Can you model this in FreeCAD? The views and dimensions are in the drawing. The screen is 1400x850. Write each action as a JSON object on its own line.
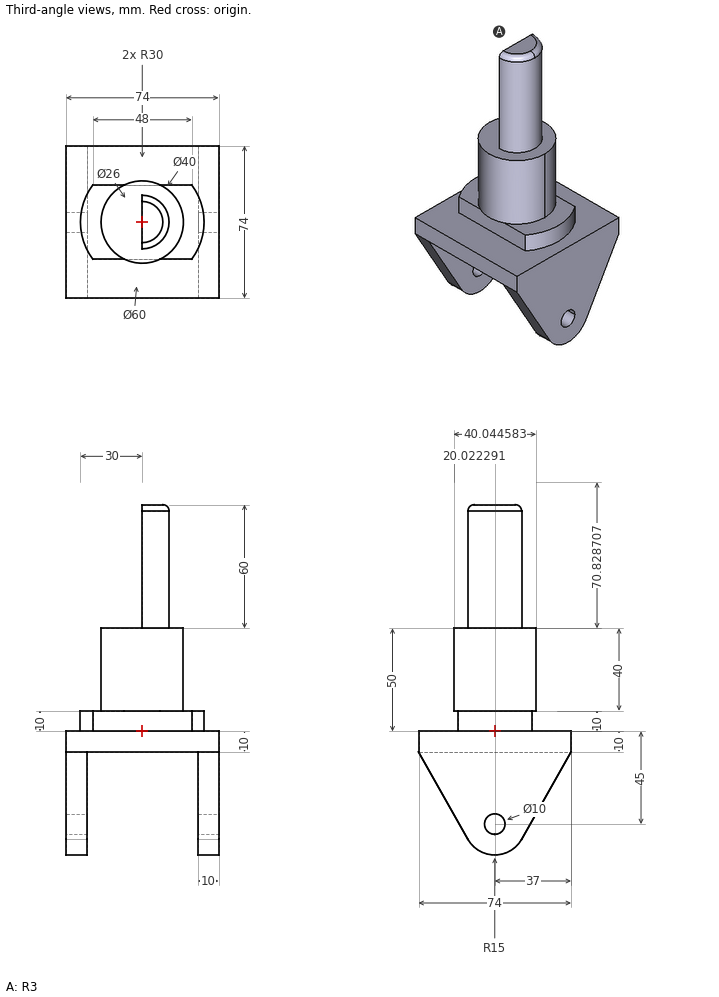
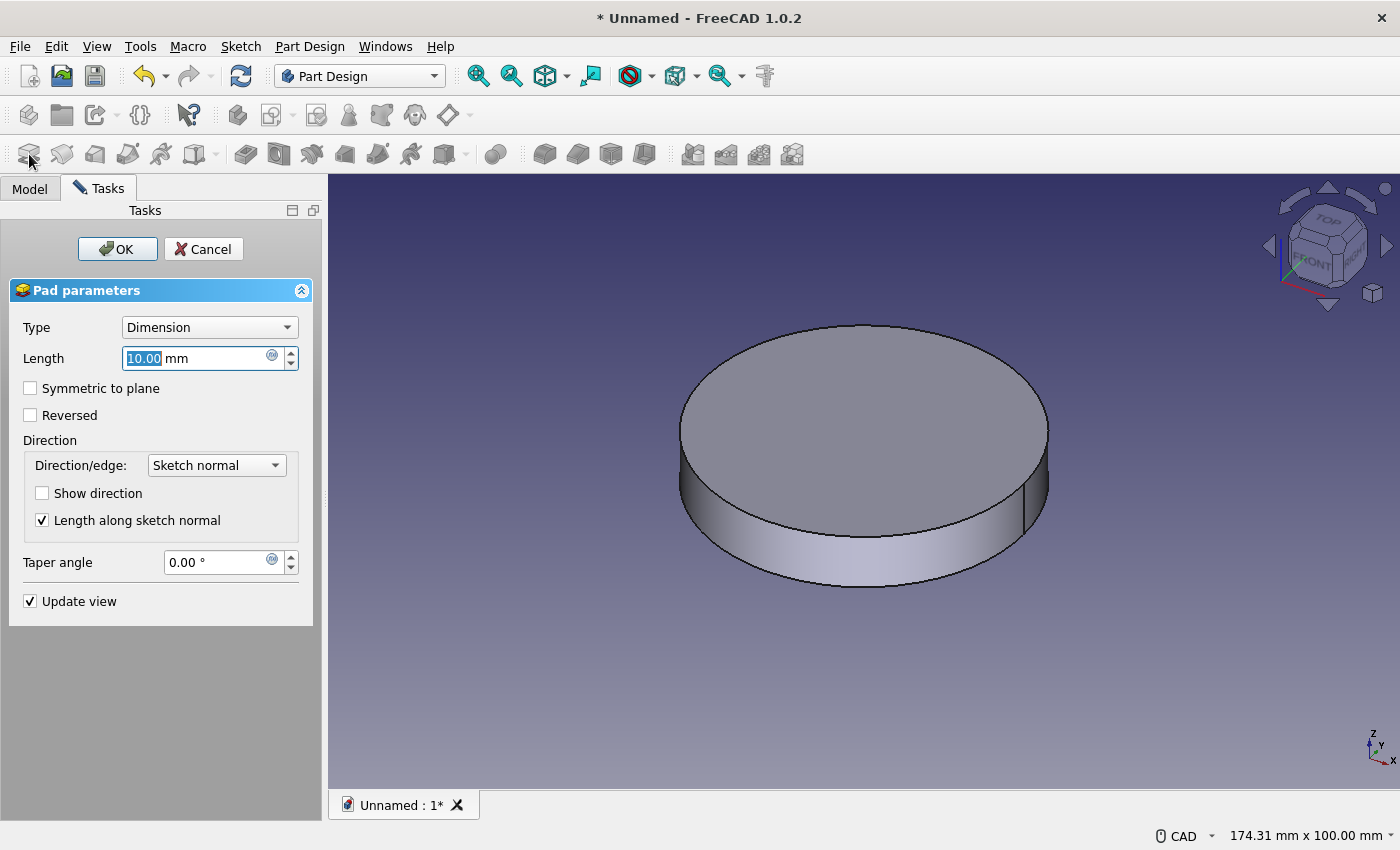
{"action": "type", "text": "10"}
{"action": "key", "text": "Tab"}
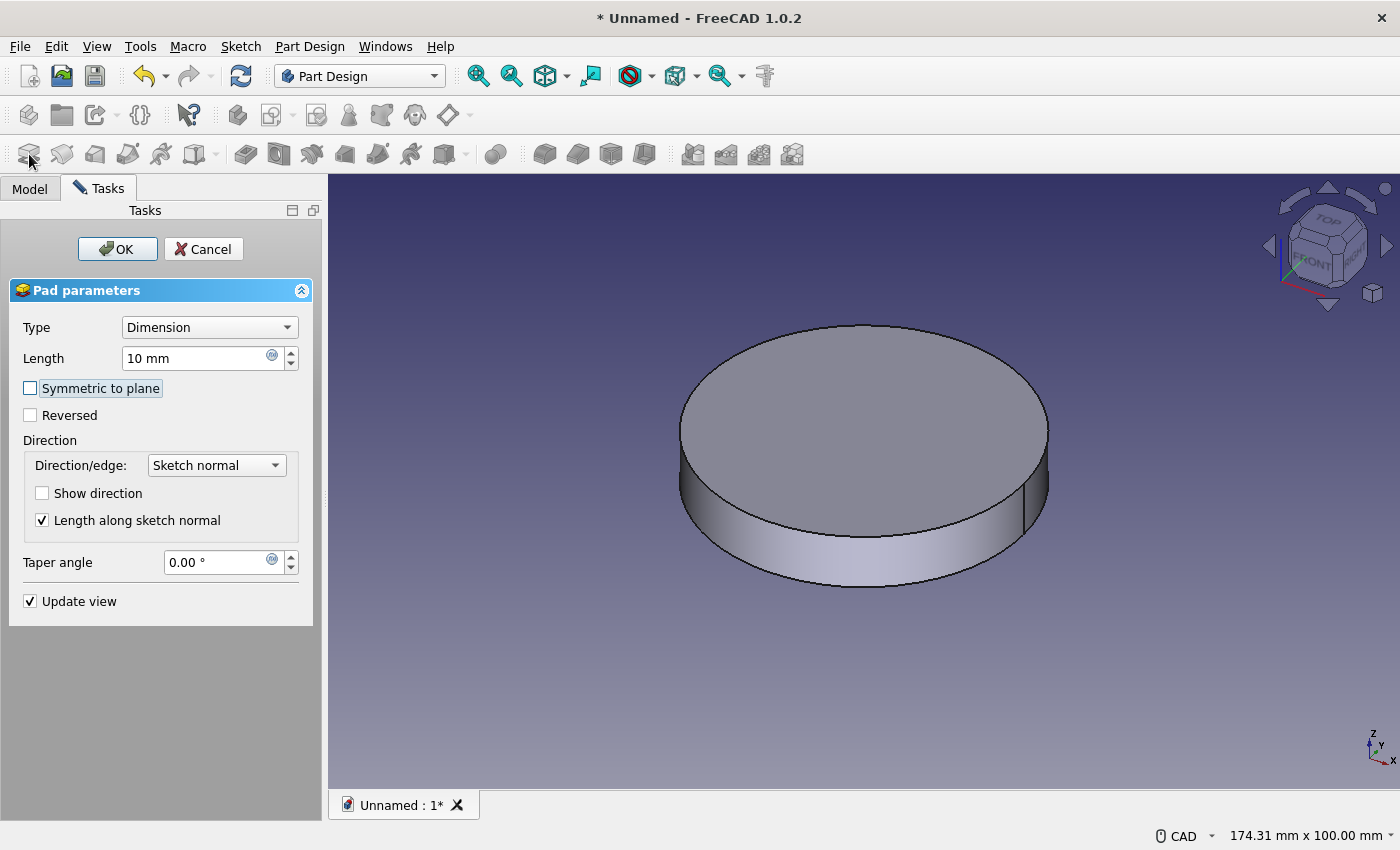
{"action": "left_click", "coordinate": [118, 249]}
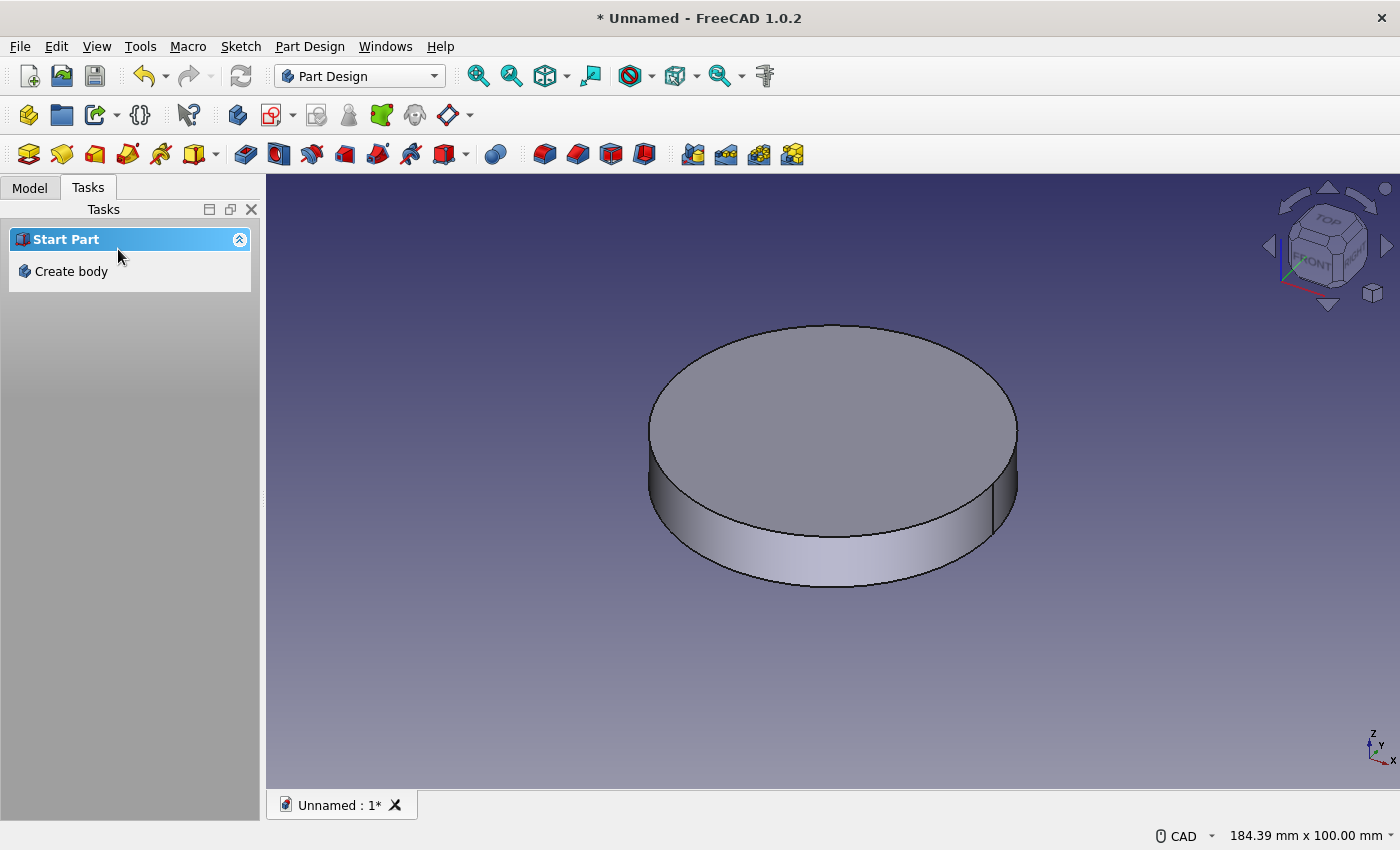
{"action": "key", "text": "5"}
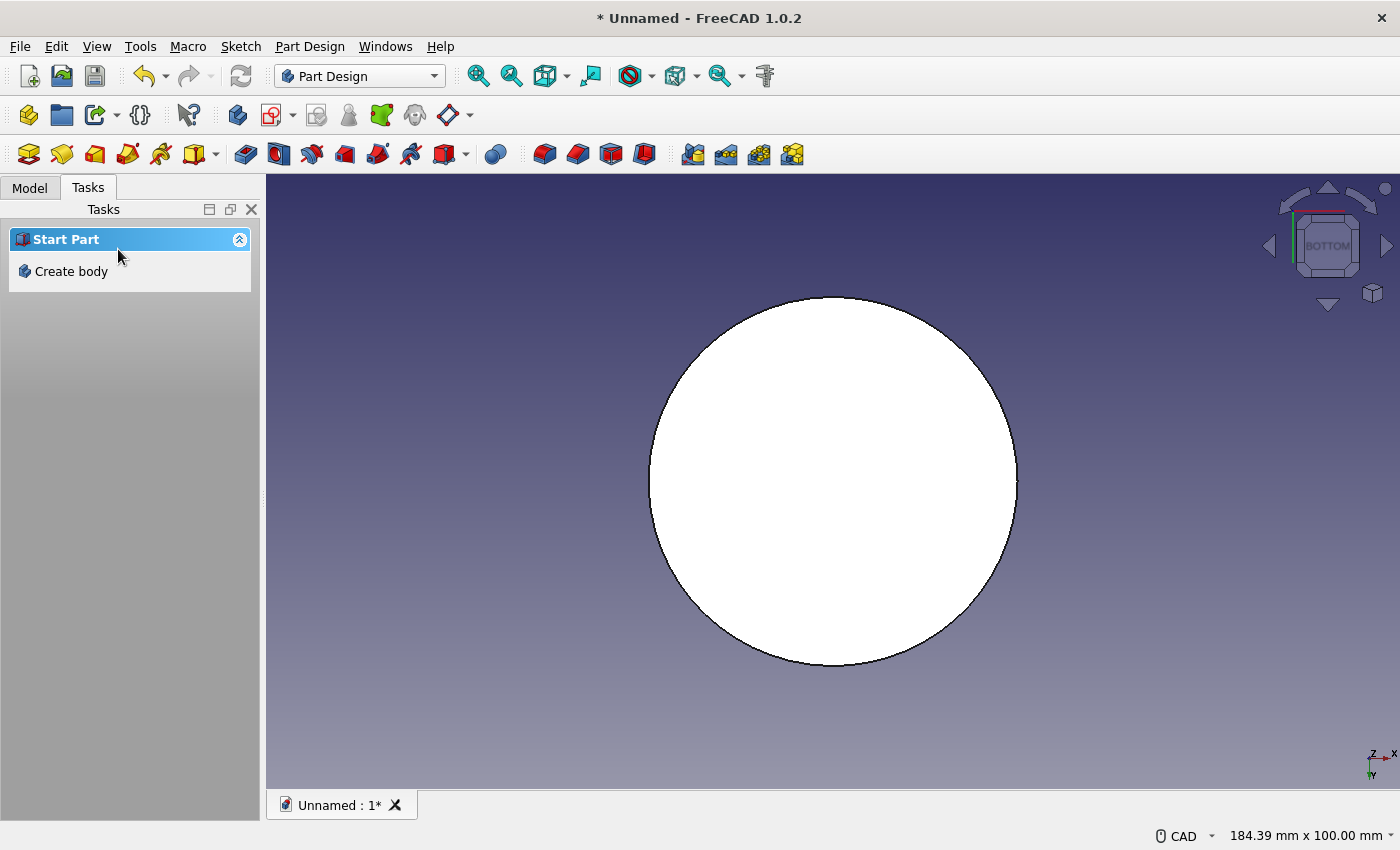
{"action": "left_click", "coordinate": [833, 480]}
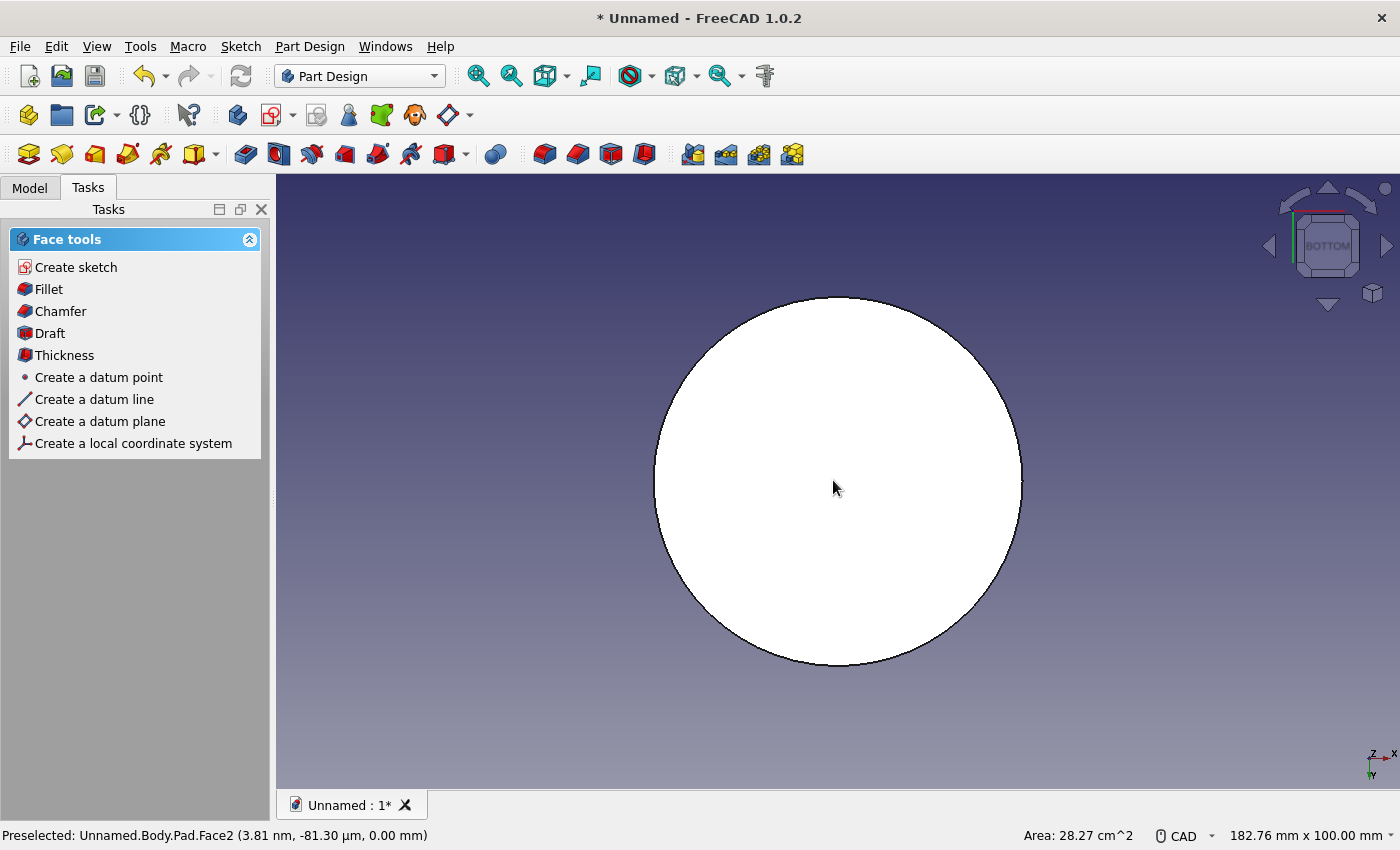
{"action": "left_click", "coordinate": [270, 116]}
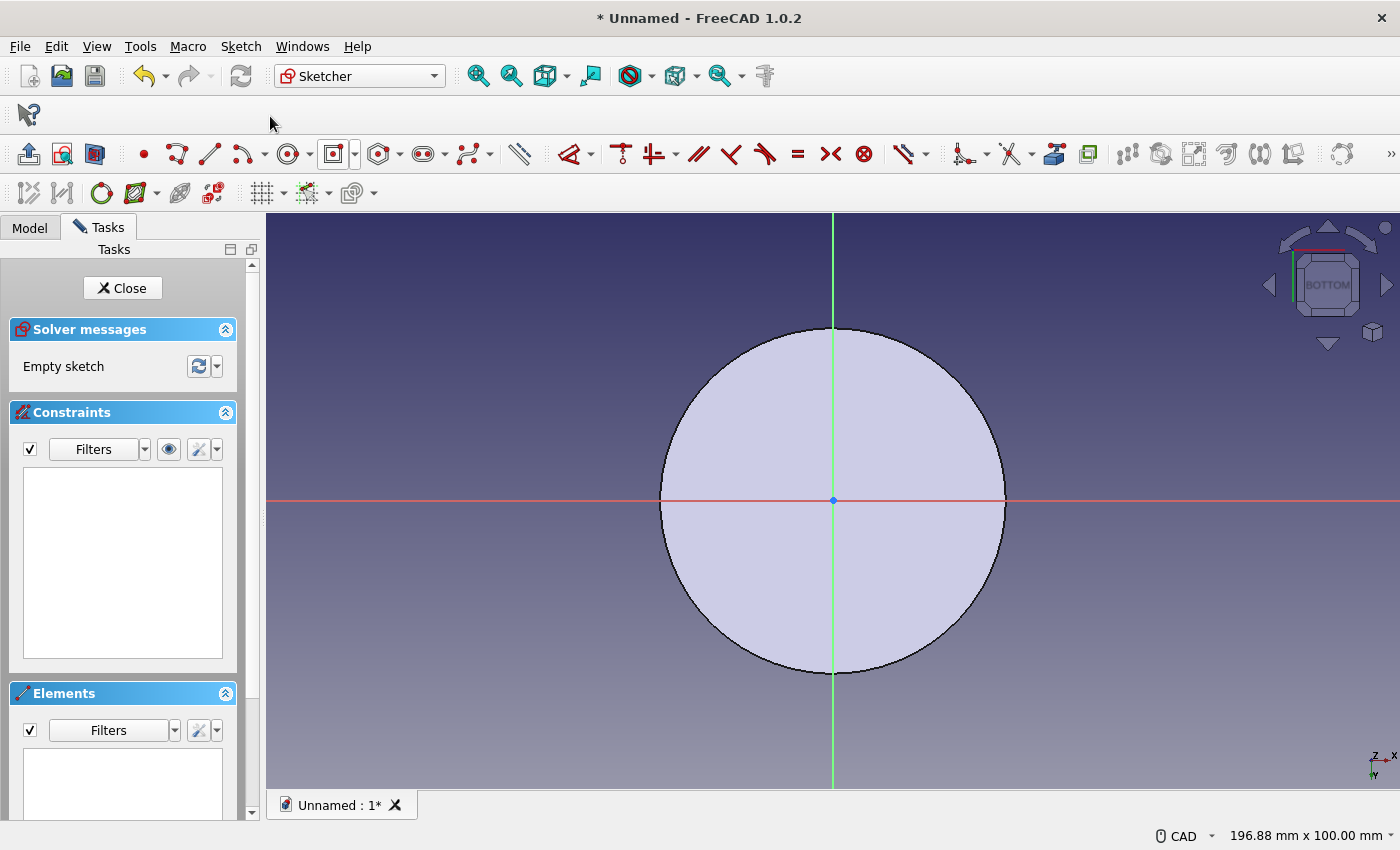
{"action": "left_click", "coordinate": [210, 154]}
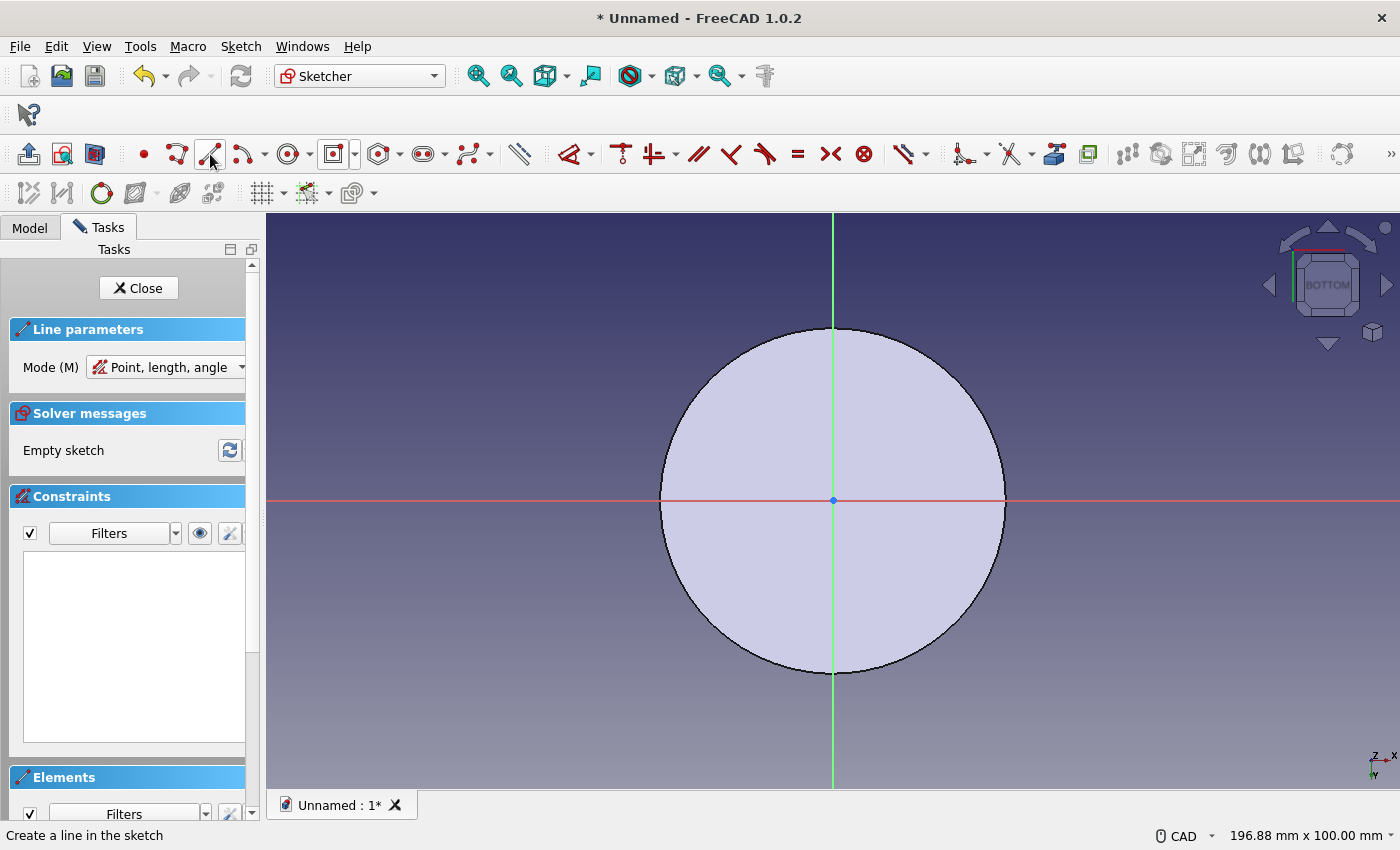
{"action": "left_click", "coordinate": [971, 605]}
{"action": "left_click", "coordinate": [695, 605]}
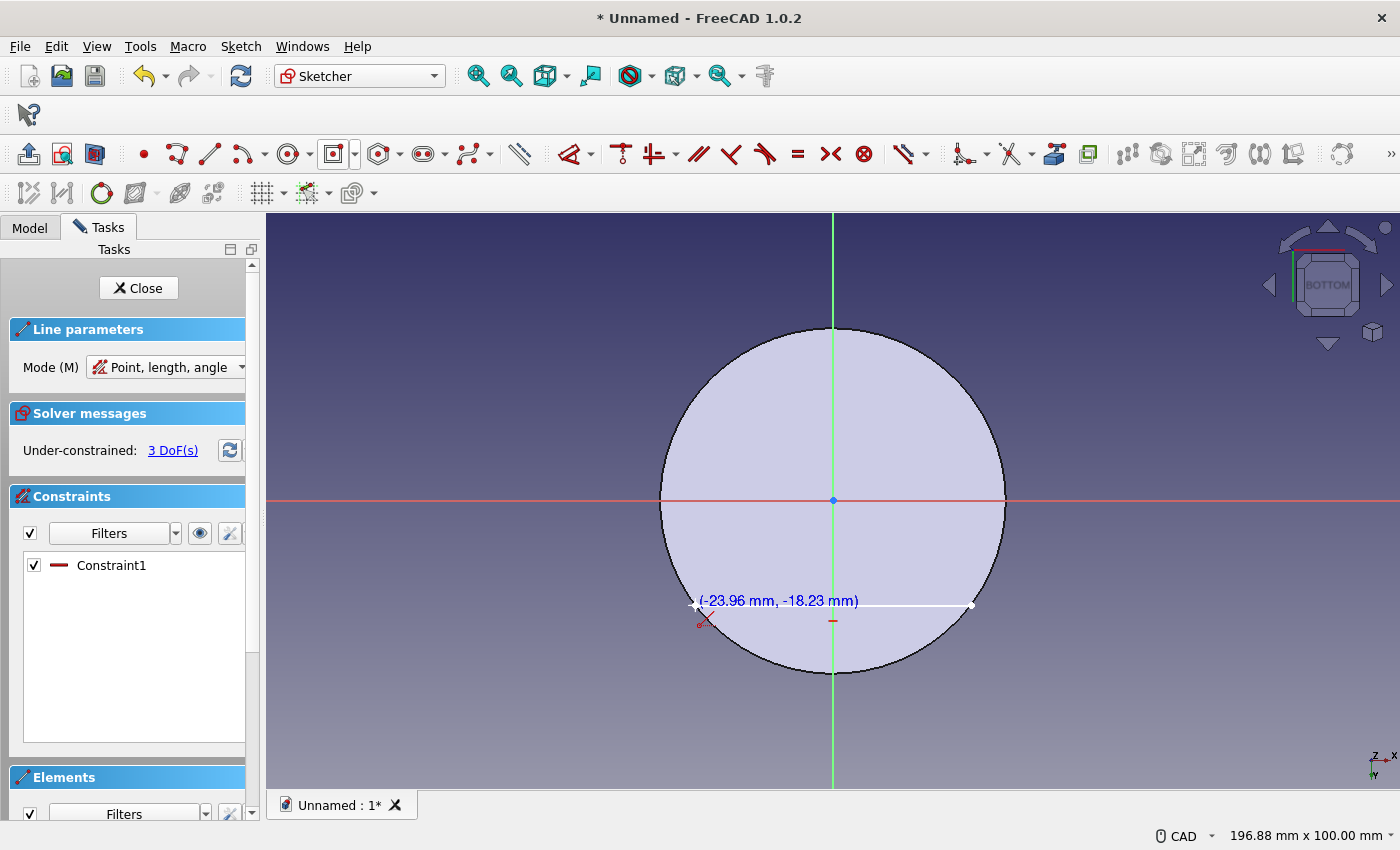
{"action": "key", "text": "g 3 a"}